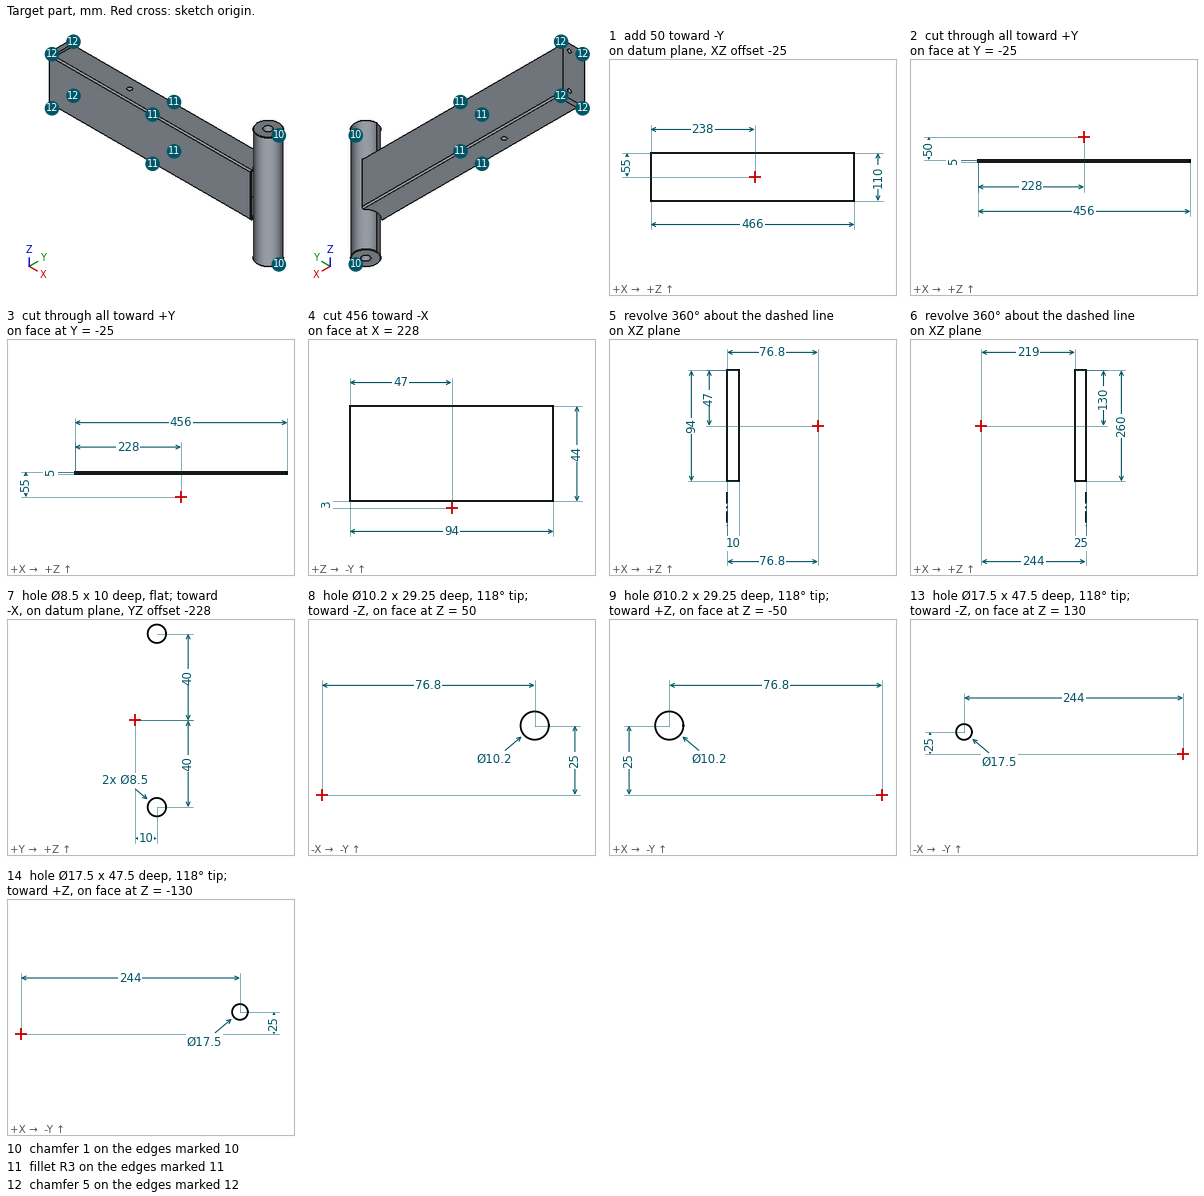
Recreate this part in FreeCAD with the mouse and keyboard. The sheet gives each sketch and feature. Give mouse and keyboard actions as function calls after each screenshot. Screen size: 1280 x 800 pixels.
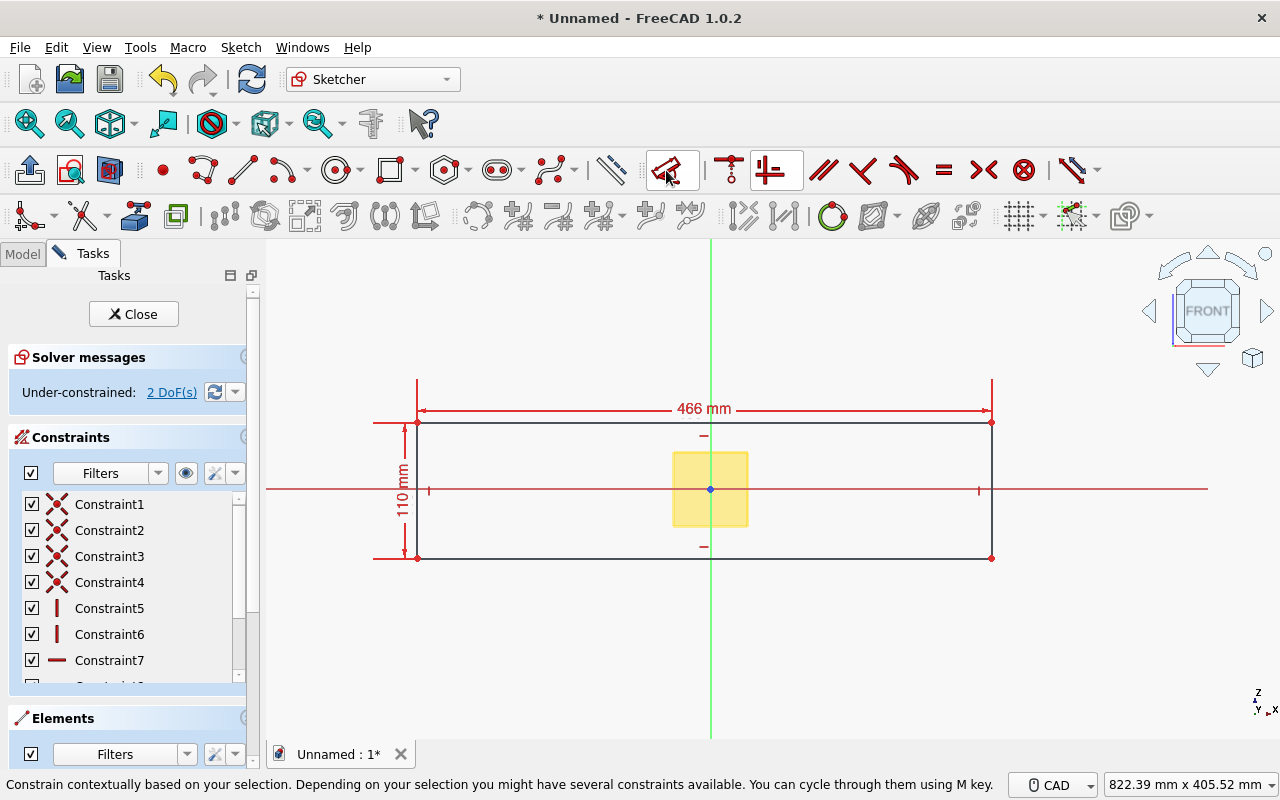
click(417, 423)
click(383, 456)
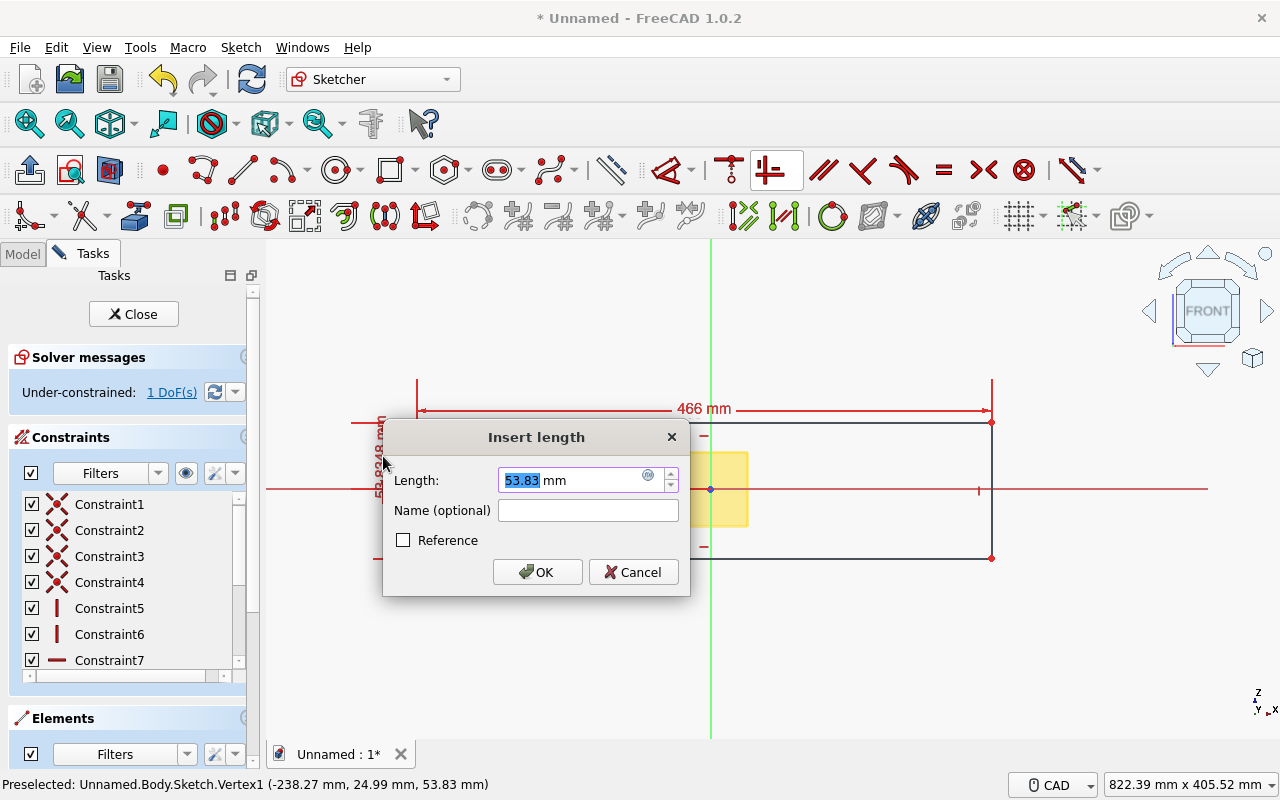
text(55)
key(Return)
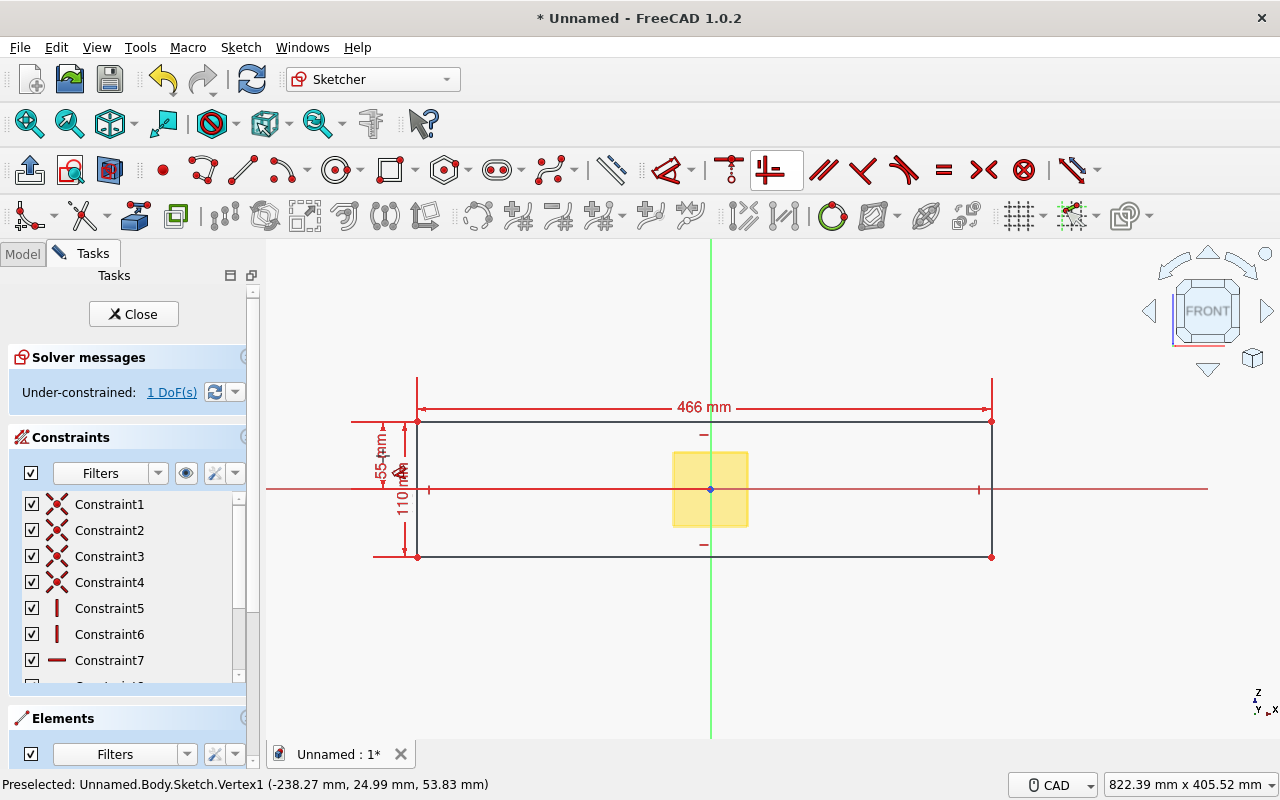
click(417, 422)
click(564, 388)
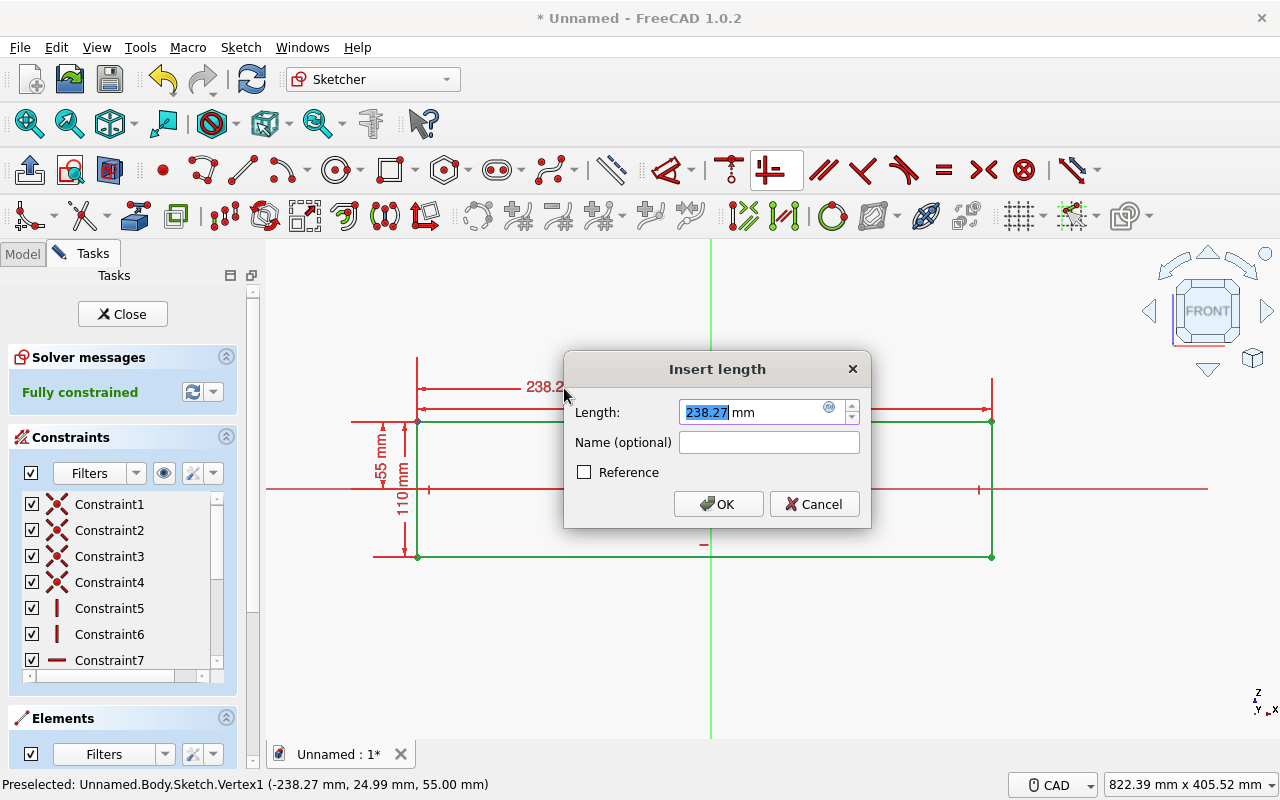
text(238)
key(Return)
key(Escape)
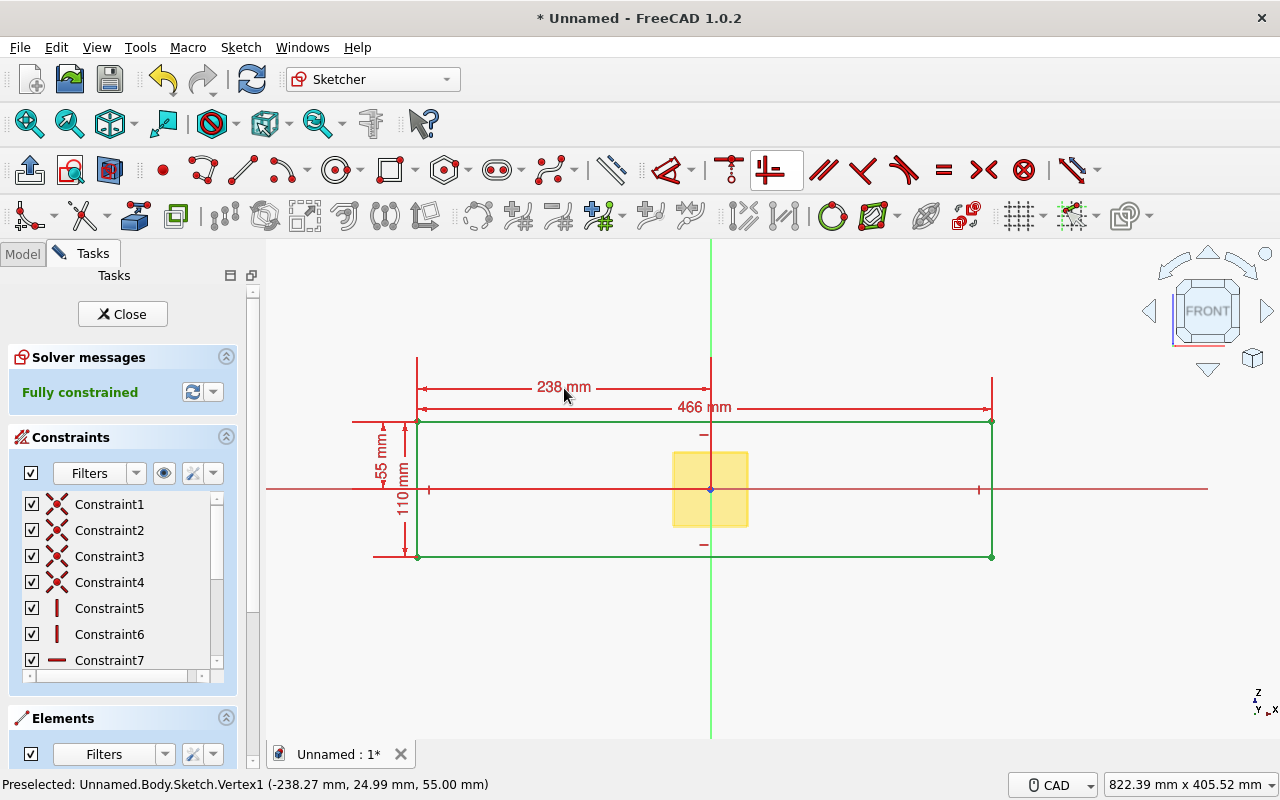
click(123, 314)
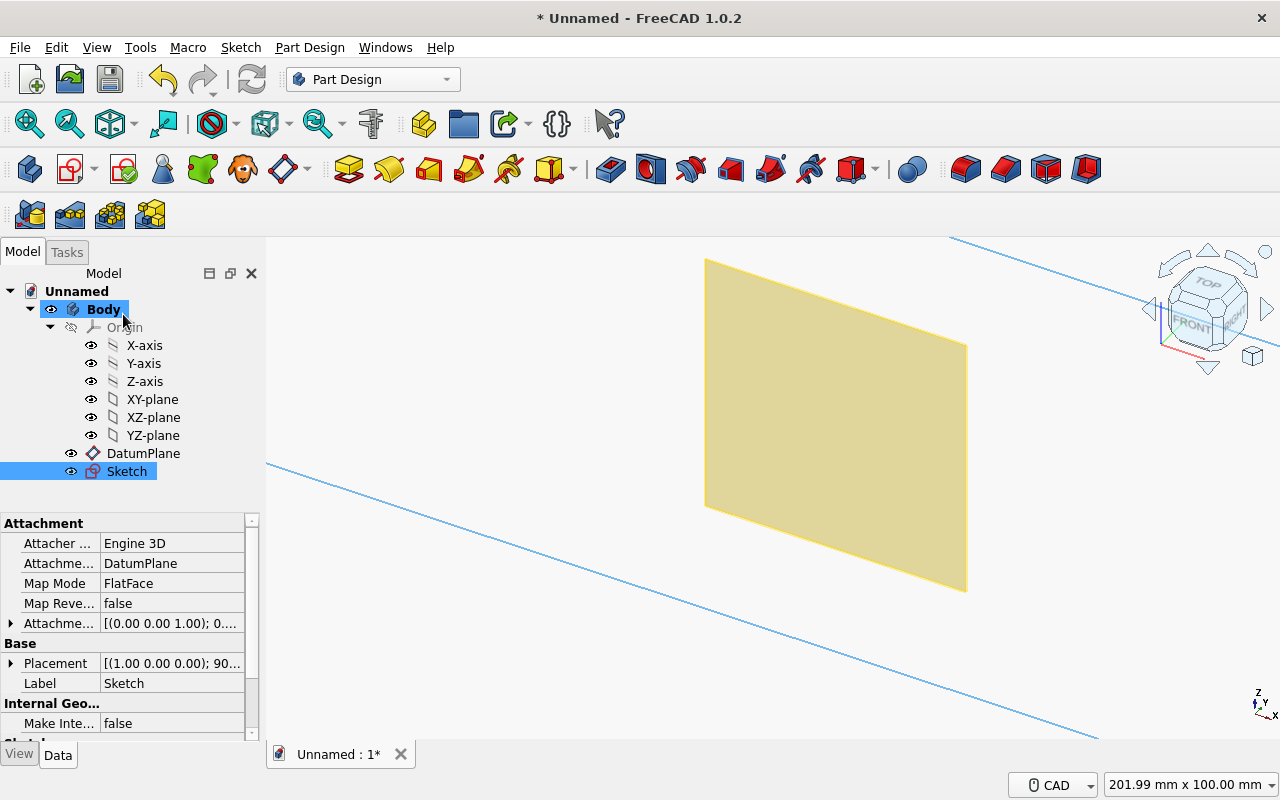
click(350, 170)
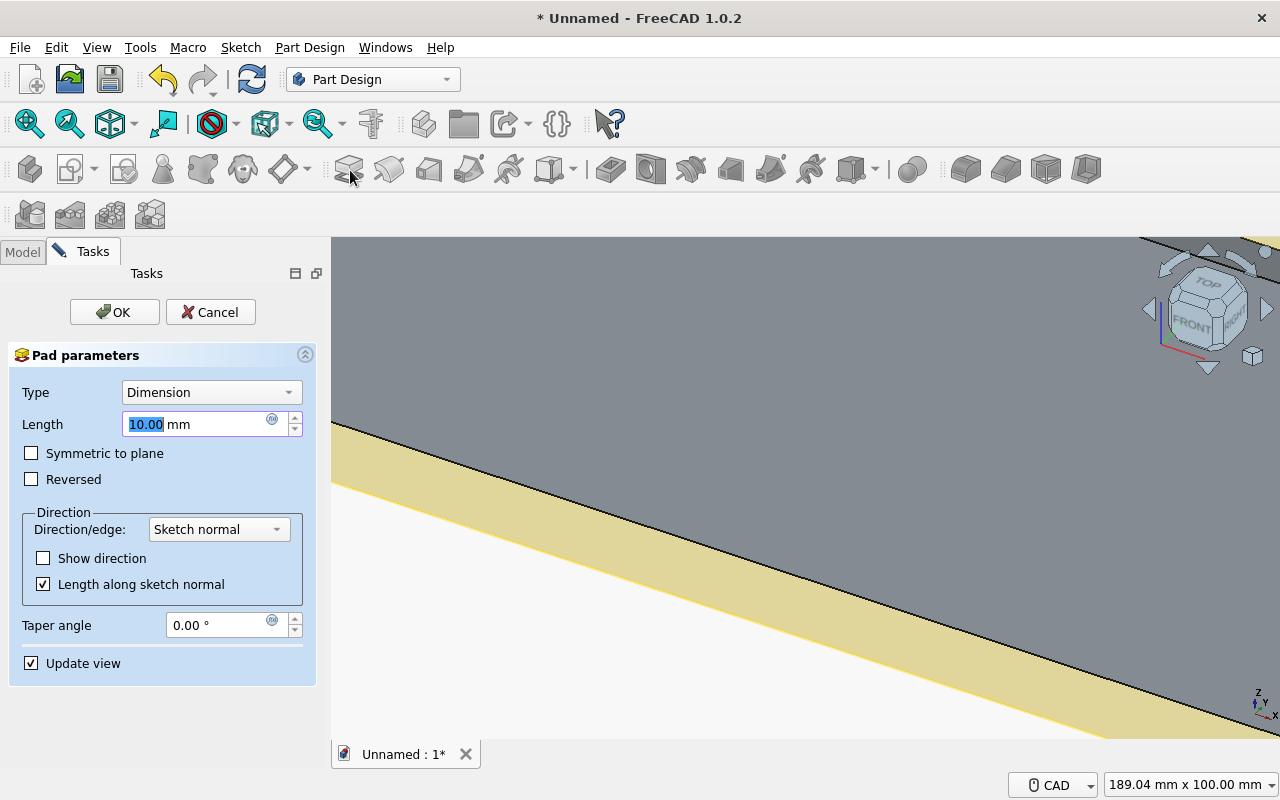
text(50)
key(Tab)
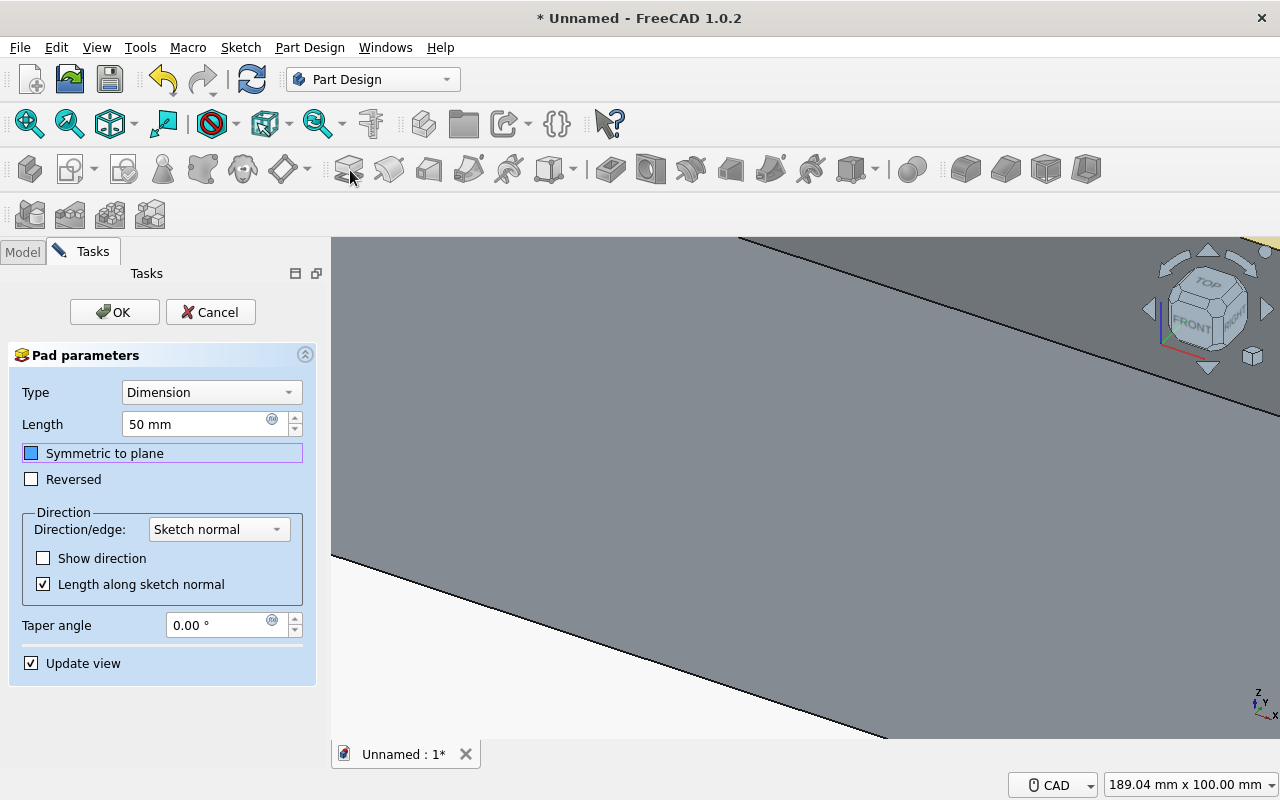
click(115, 312)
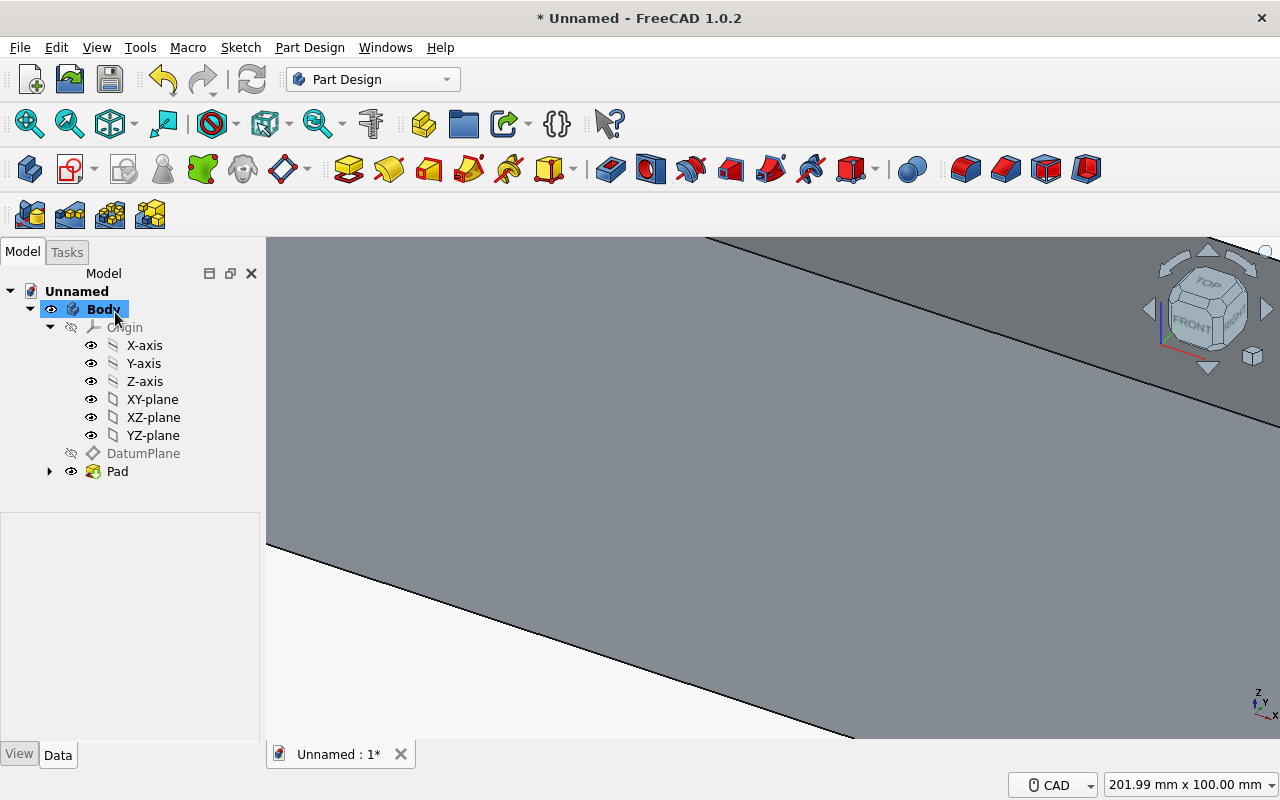
click(30, 124)